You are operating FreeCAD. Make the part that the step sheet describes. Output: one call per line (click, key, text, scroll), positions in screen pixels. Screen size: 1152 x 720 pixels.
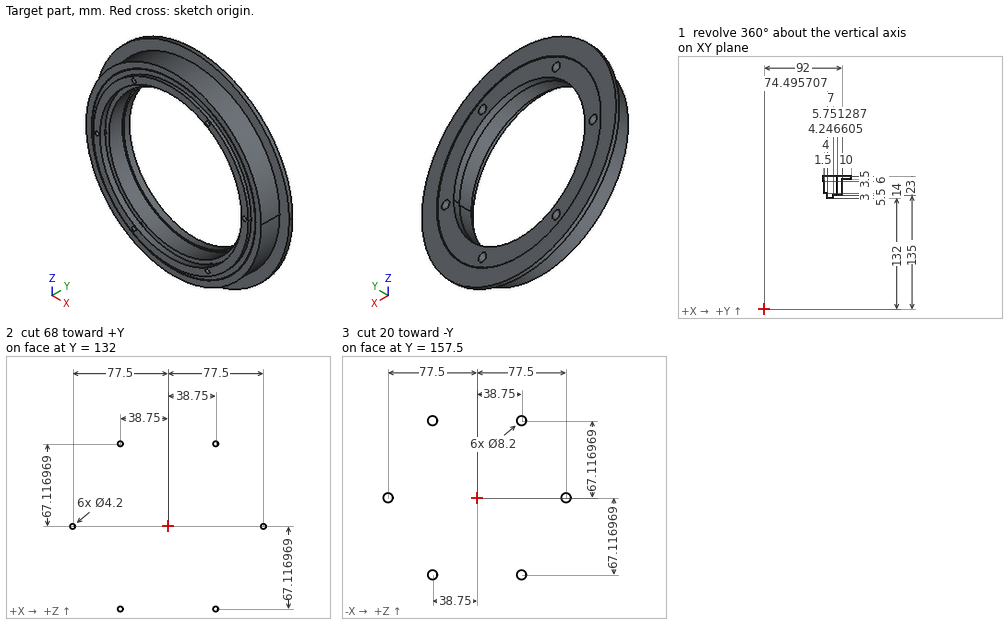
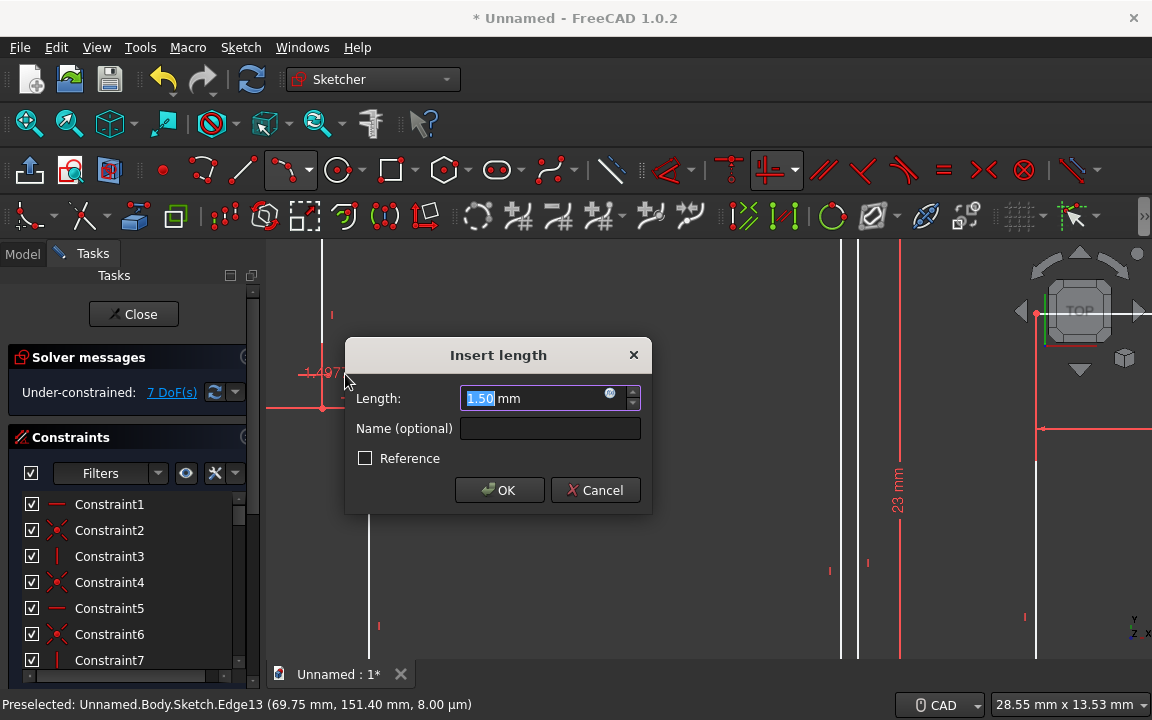
text(1.5)
key(Return)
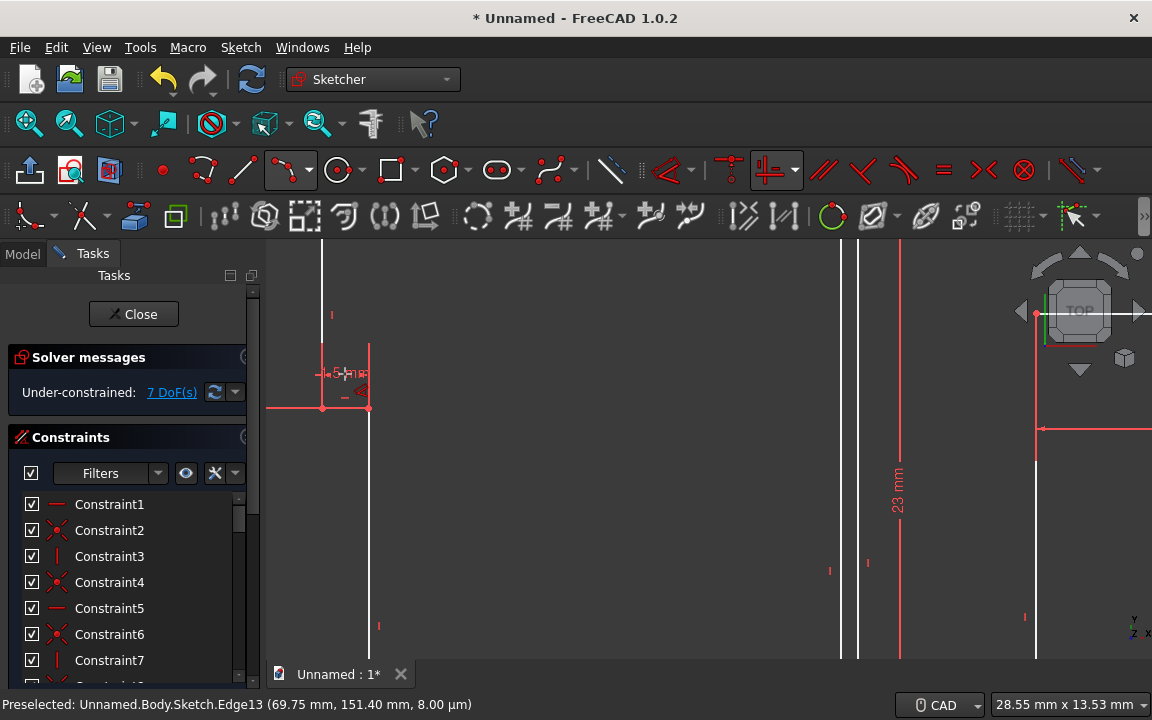
scroll(557, 381, down, 6)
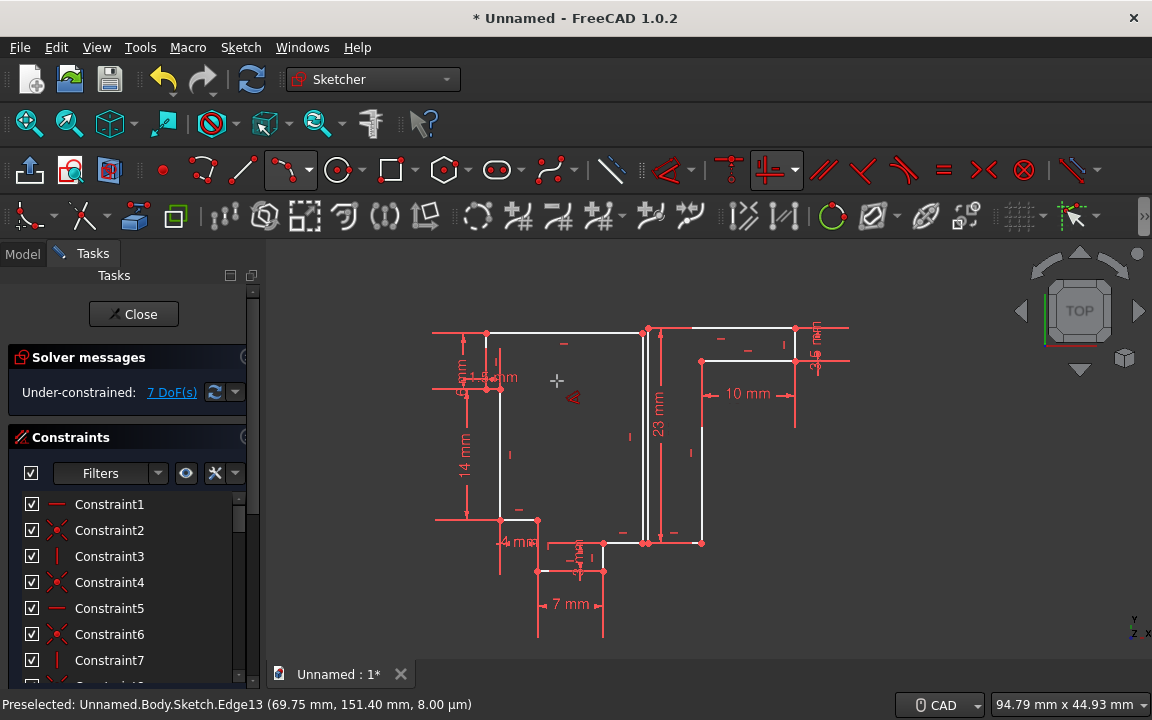
click(538, 536)
click(504, 564)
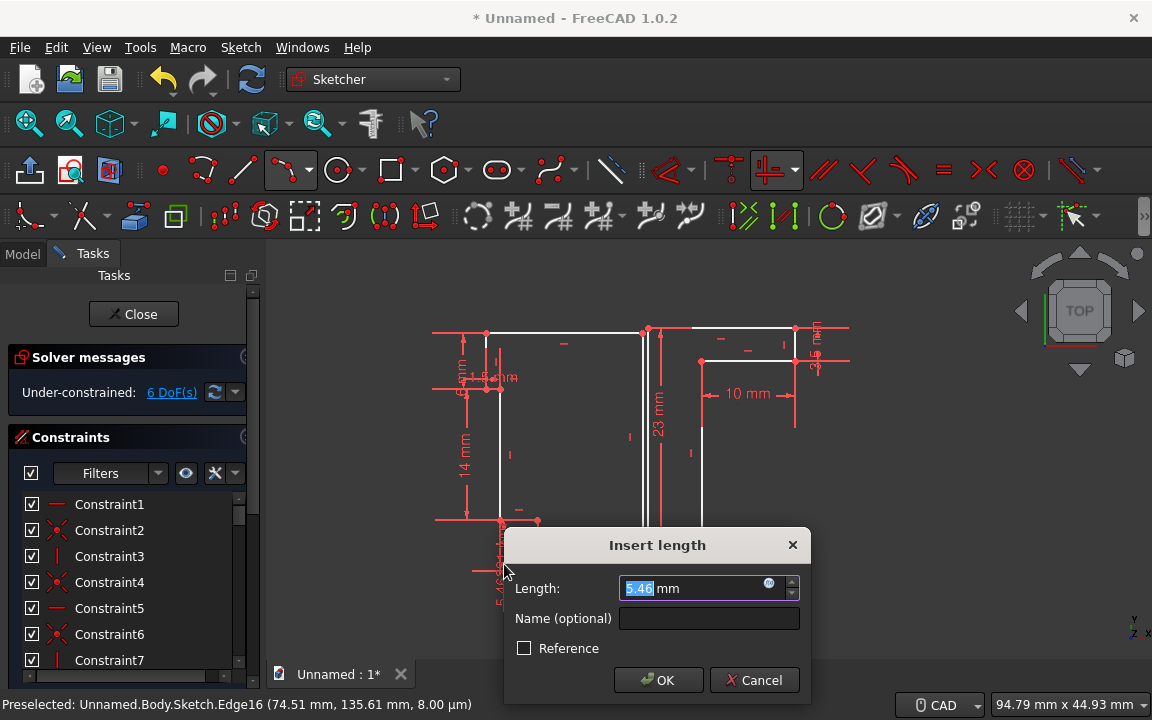
text(5.5)
key(Return)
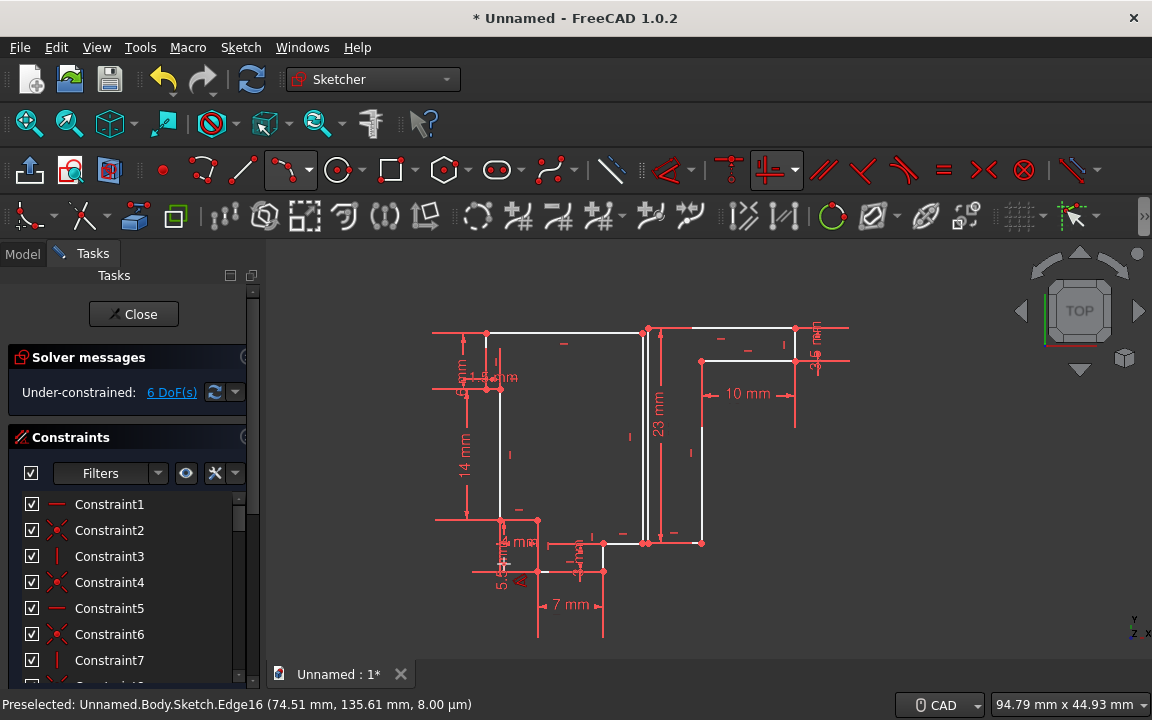
click(702, 543)
click(404, 509)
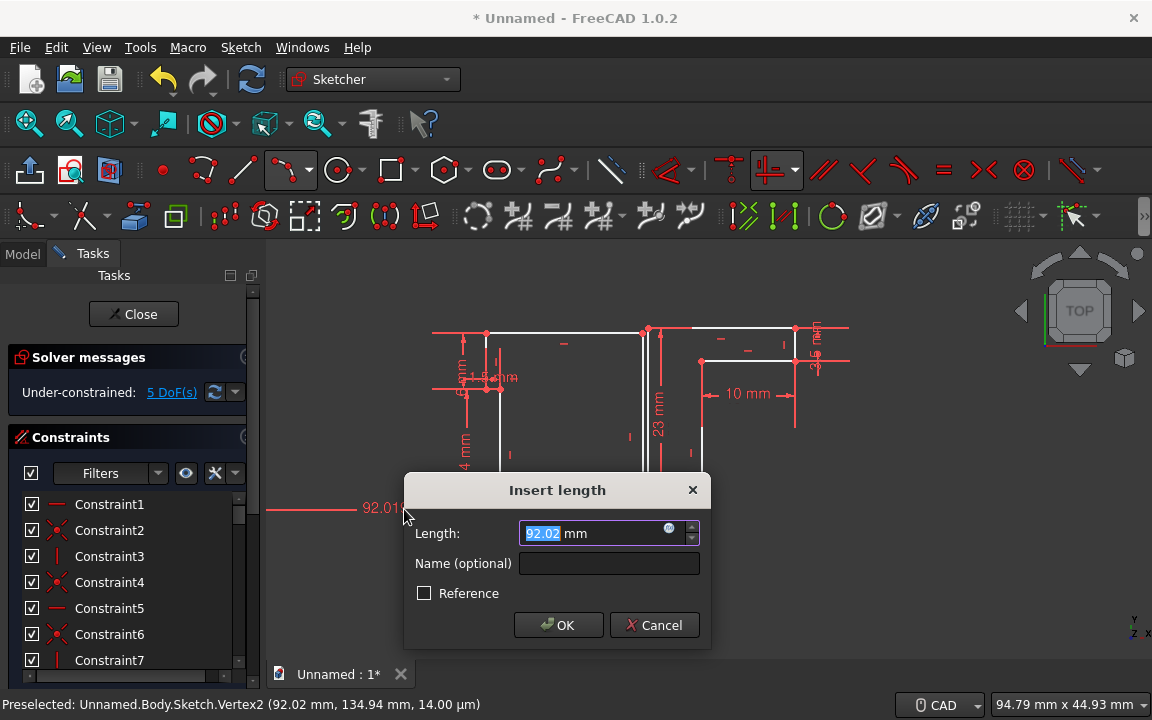
text(92)
key(Return)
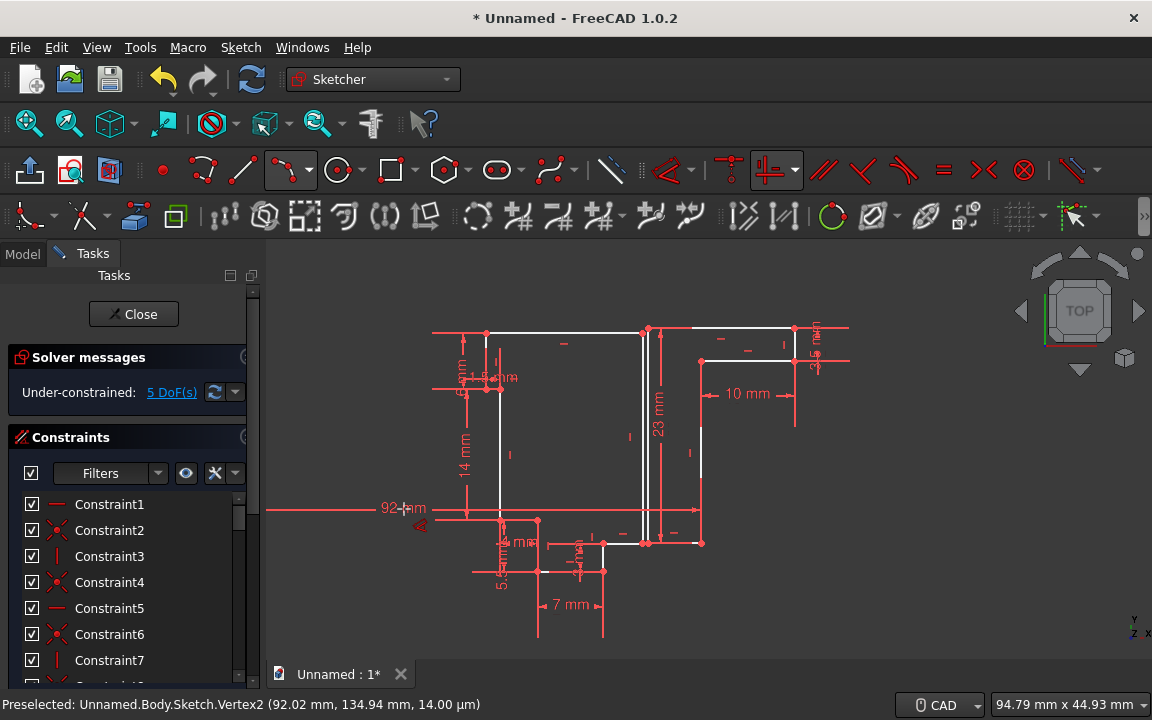
scroll(648, 543, up, 5)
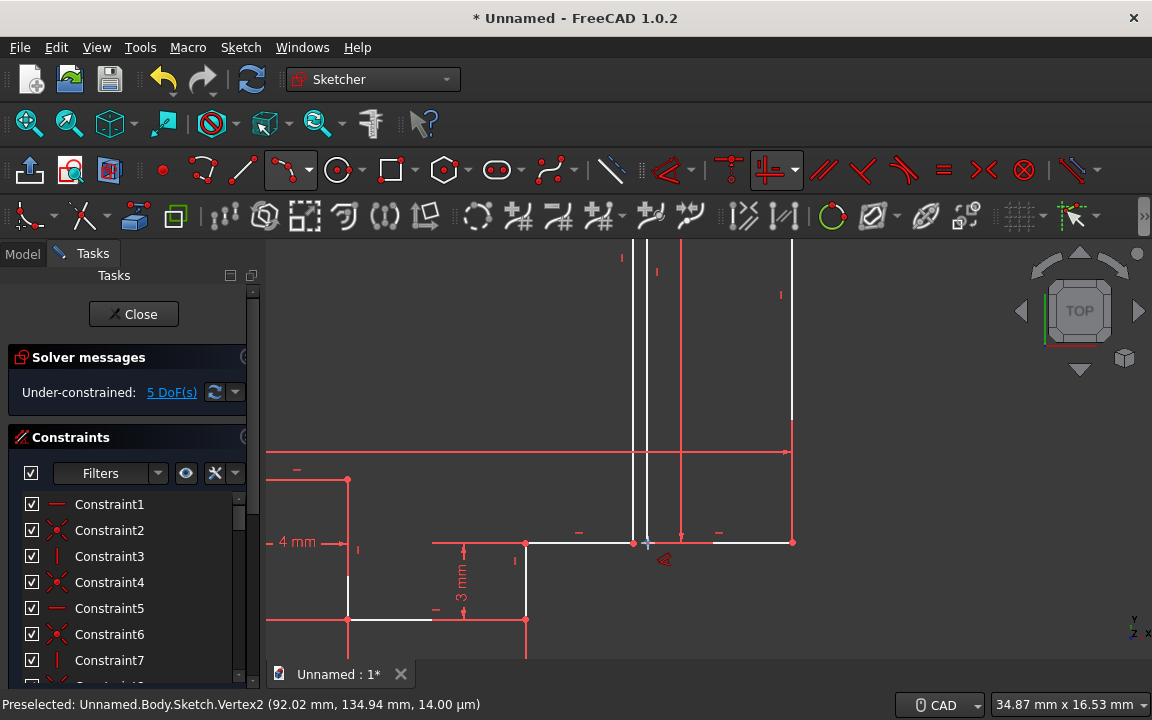
click(647, 543)
click(681, 587)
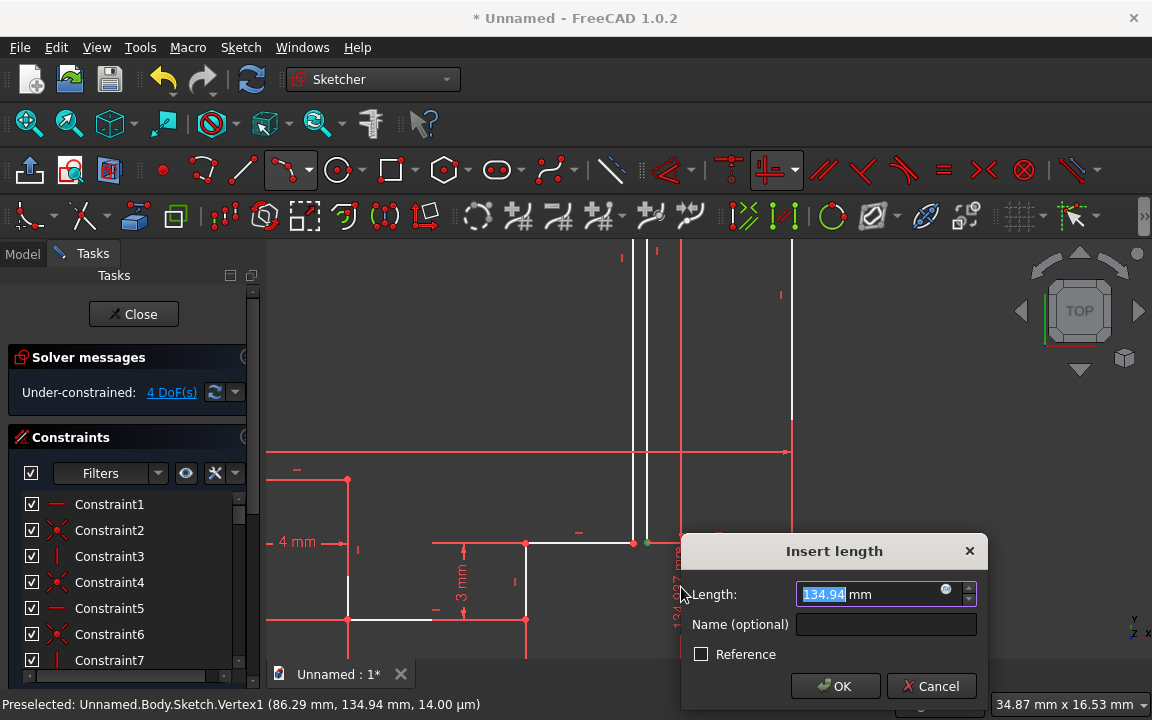
text(135)
key(Return)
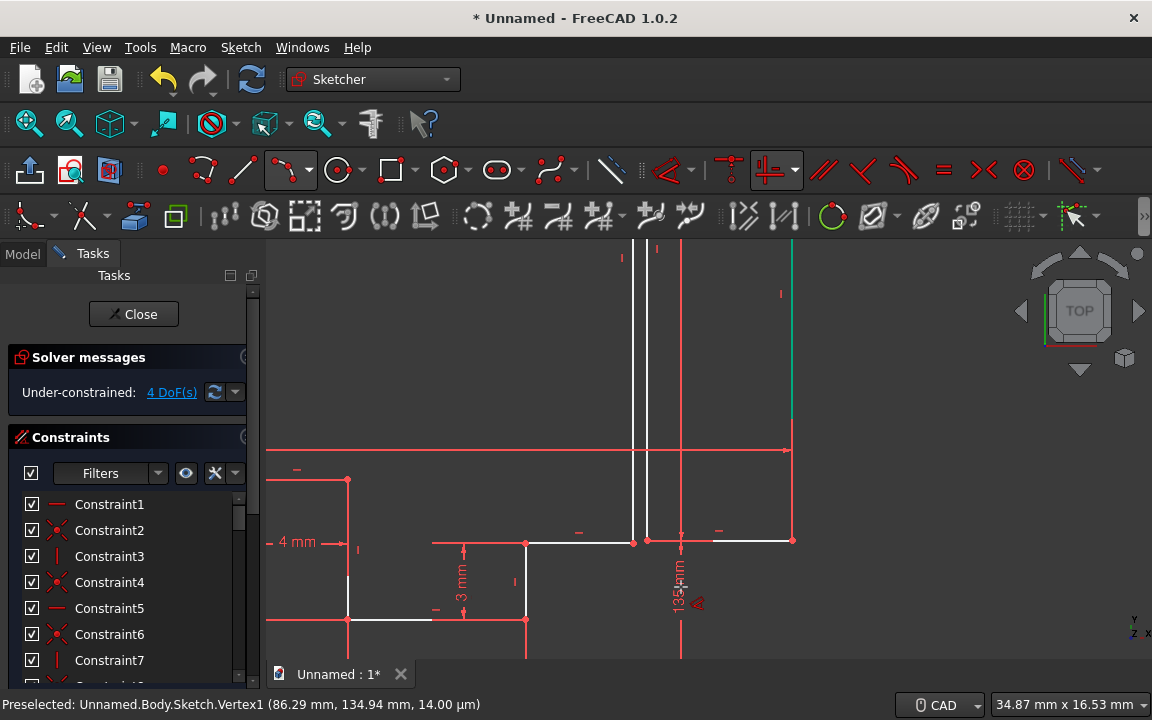
click(348, 620)
click(382, 628)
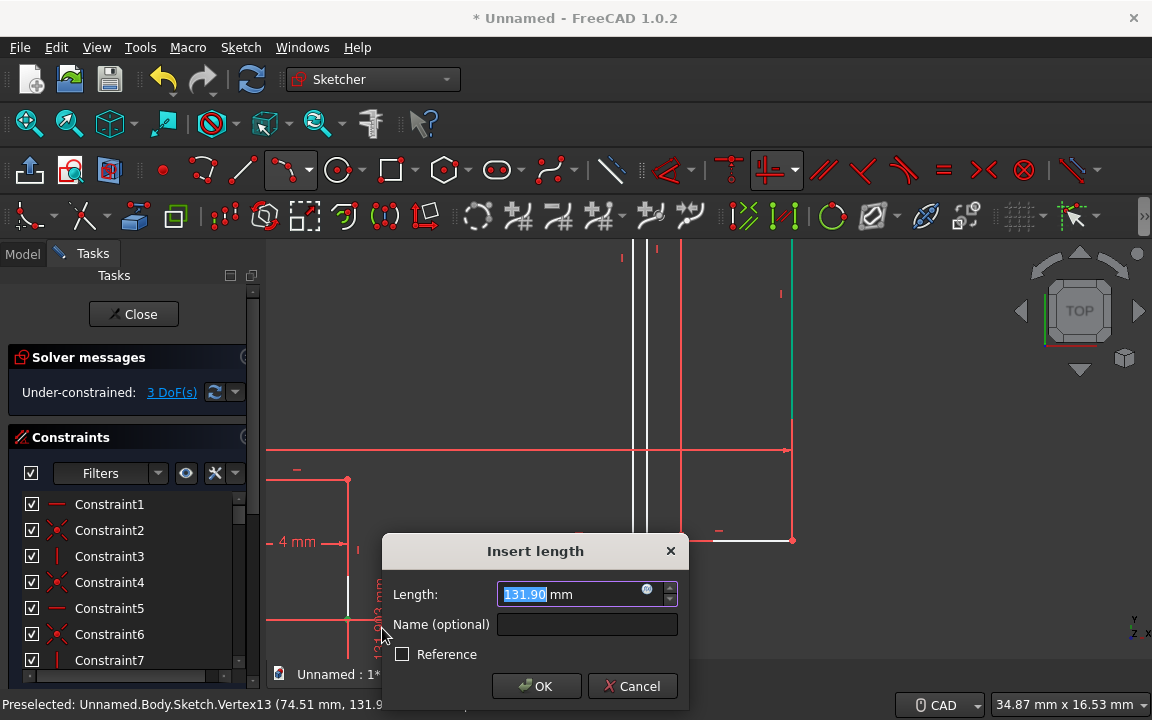
text(132)
key(Return)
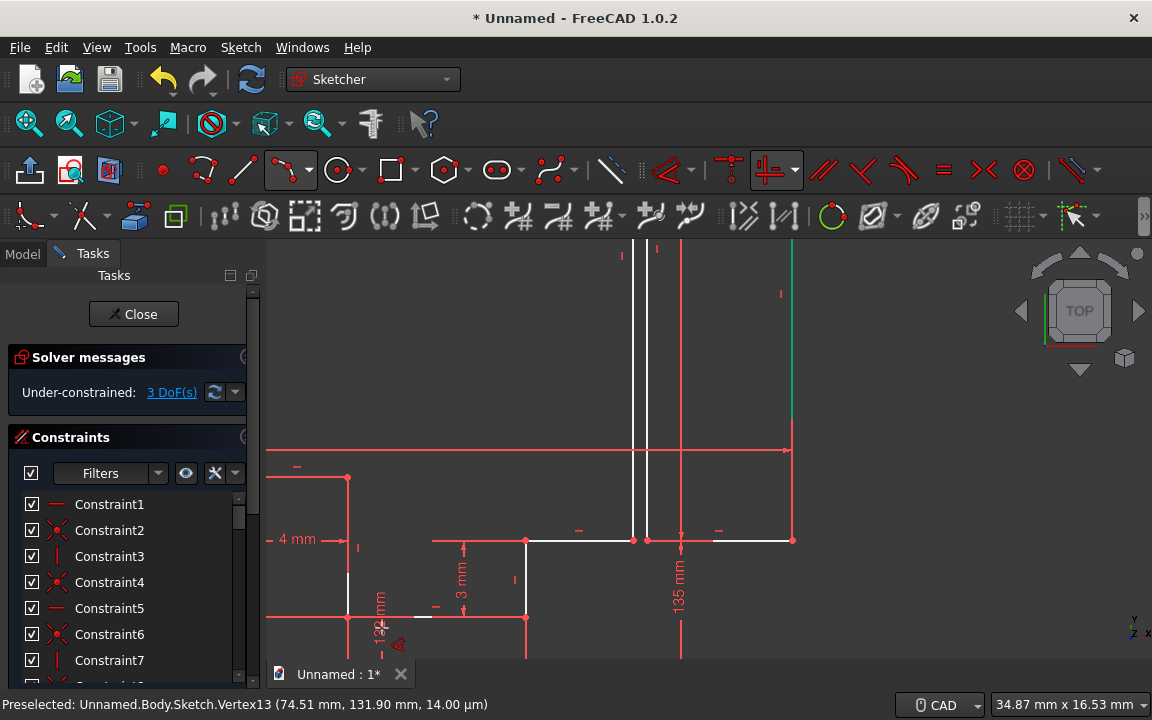
click(691, 541)
click(753, 575)